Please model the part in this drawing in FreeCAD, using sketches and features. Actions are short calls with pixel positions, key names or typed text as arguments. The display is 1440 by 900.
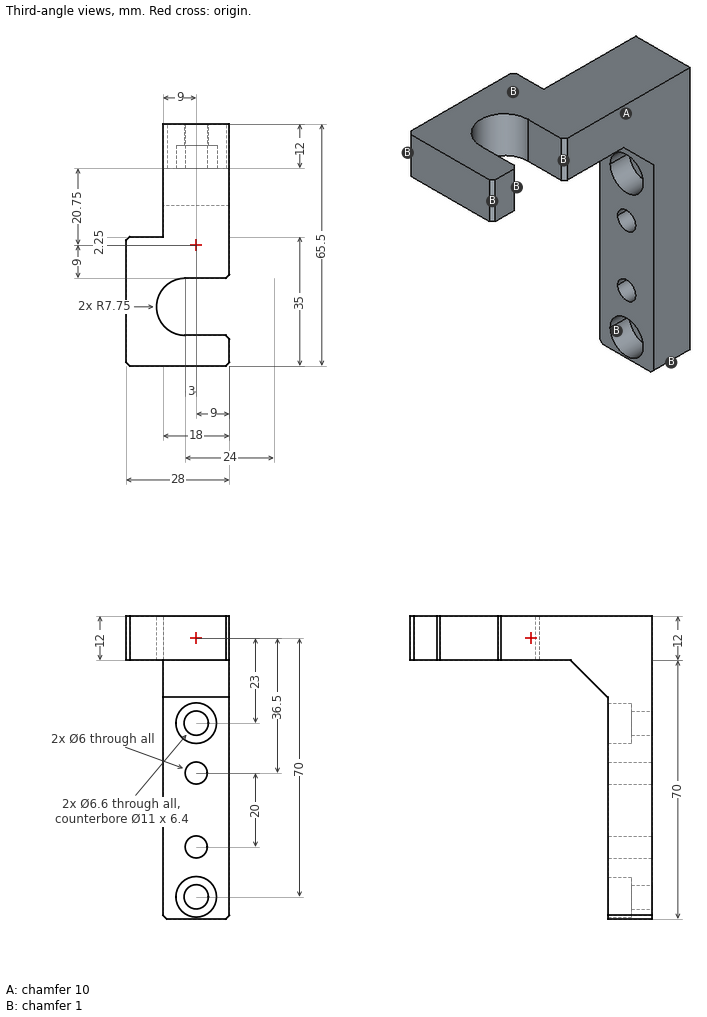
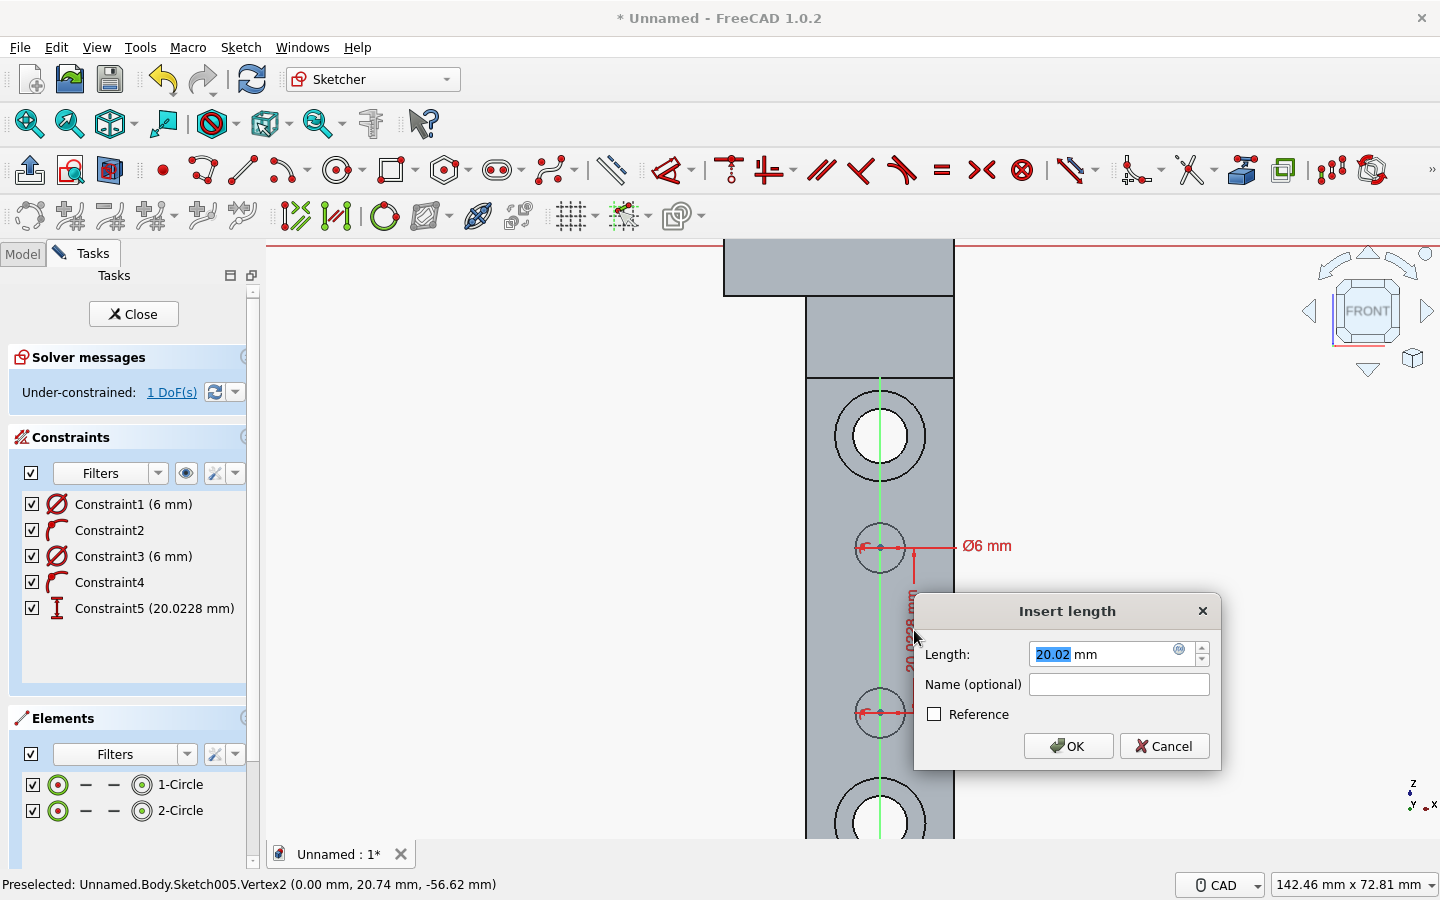
text(20)
key(Return)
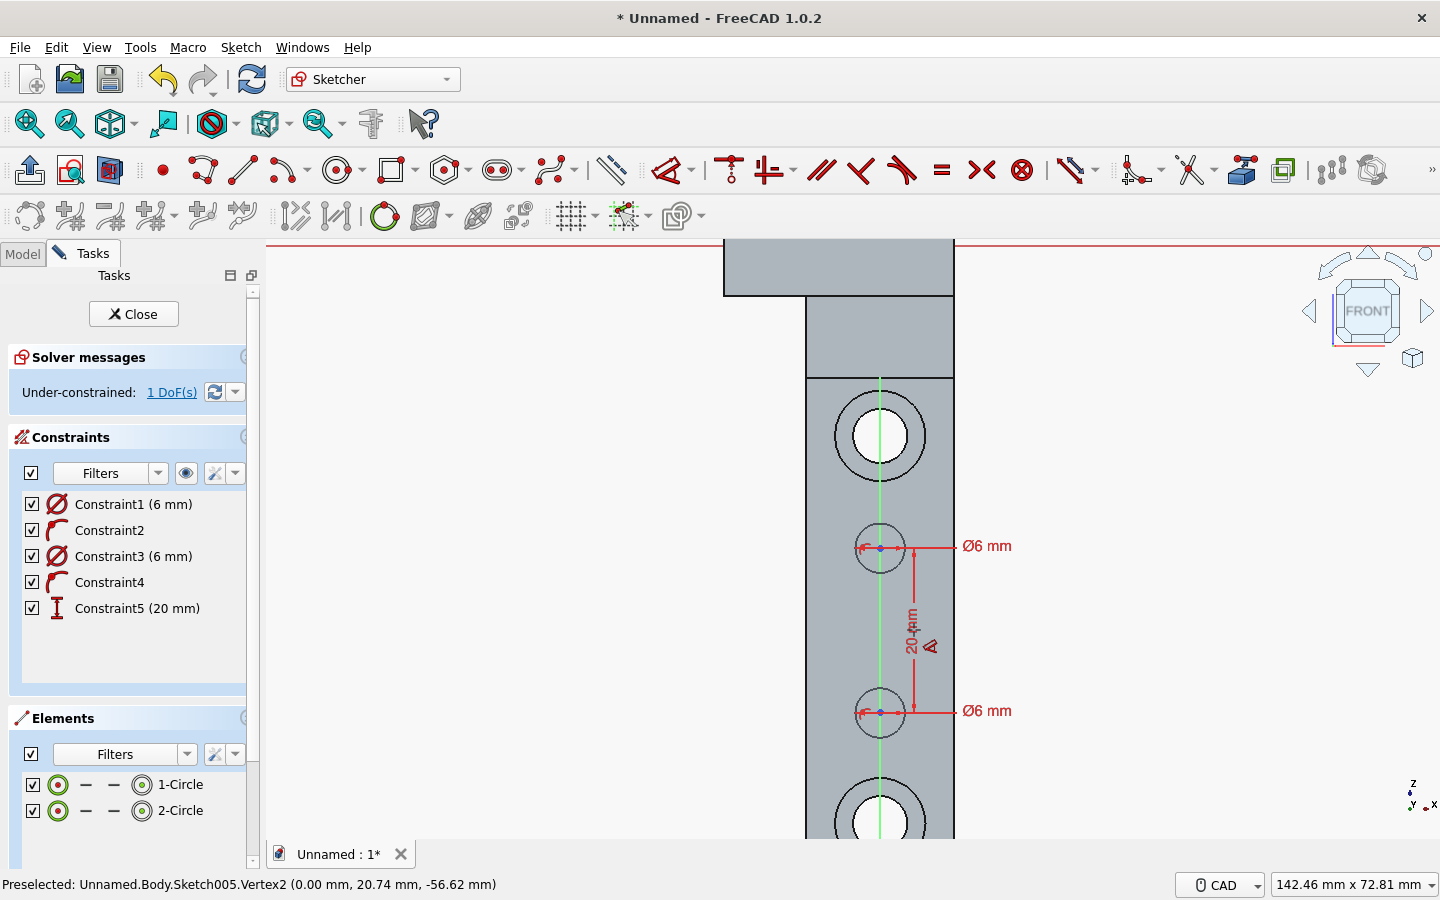
click(880, 548)
click(914, 408)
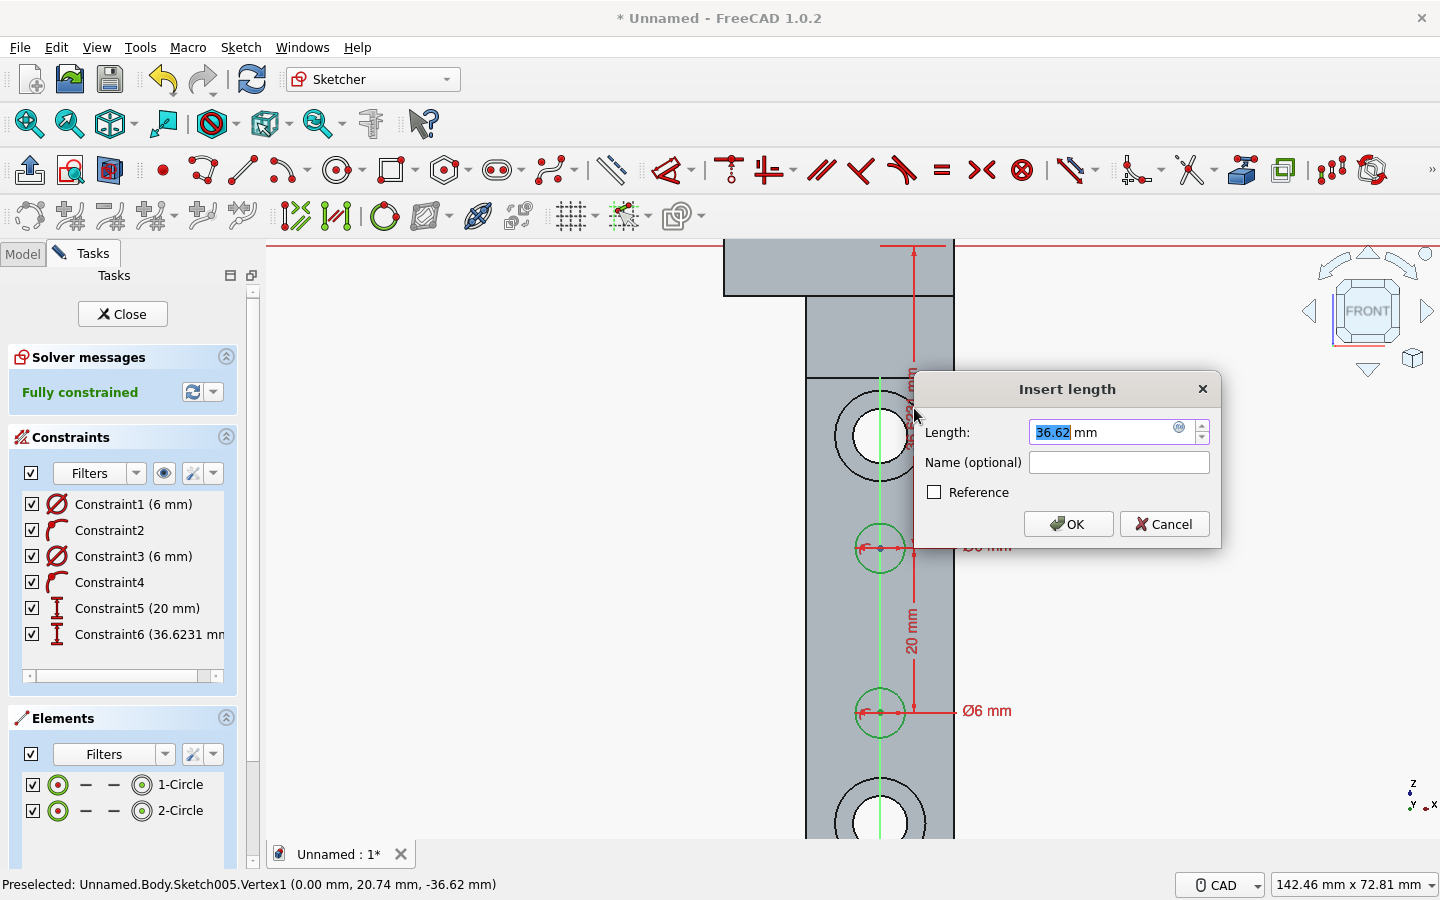
text(36.5)
key(Return)
key(Escape)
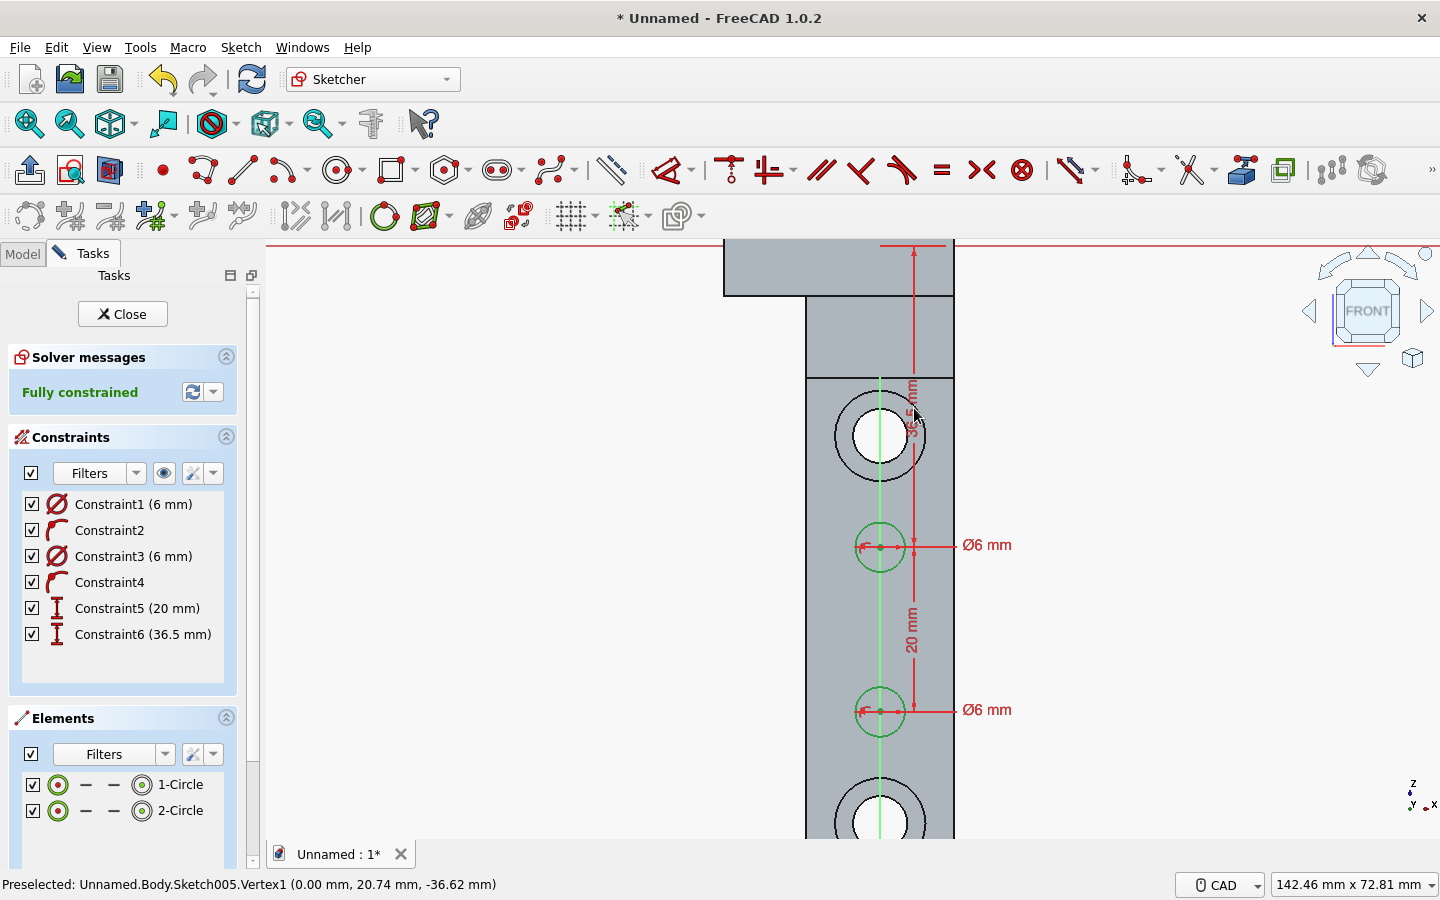
click(123, 314)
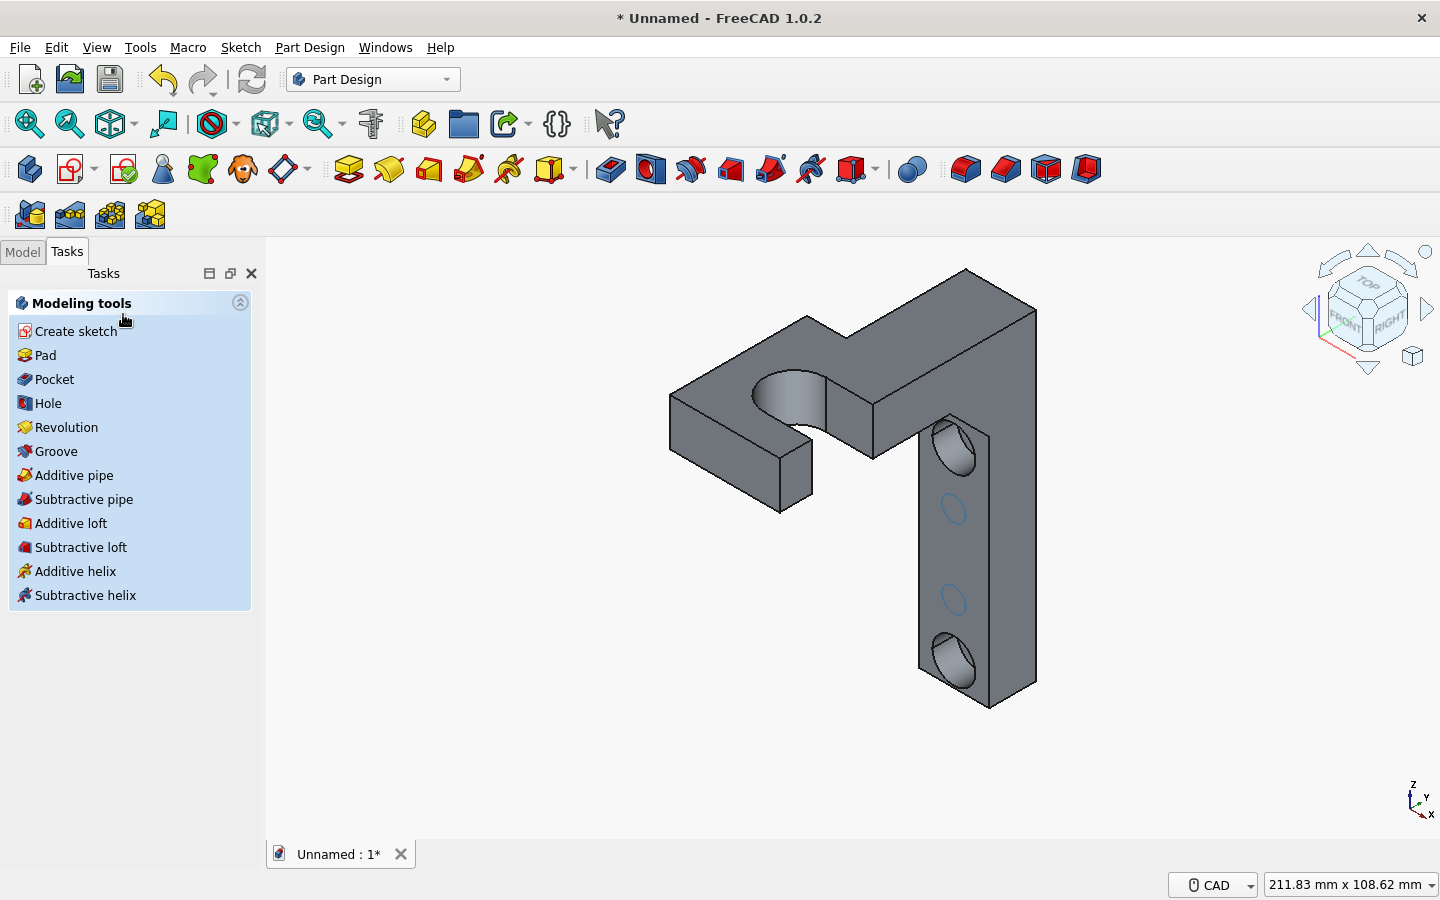
click(652, 170)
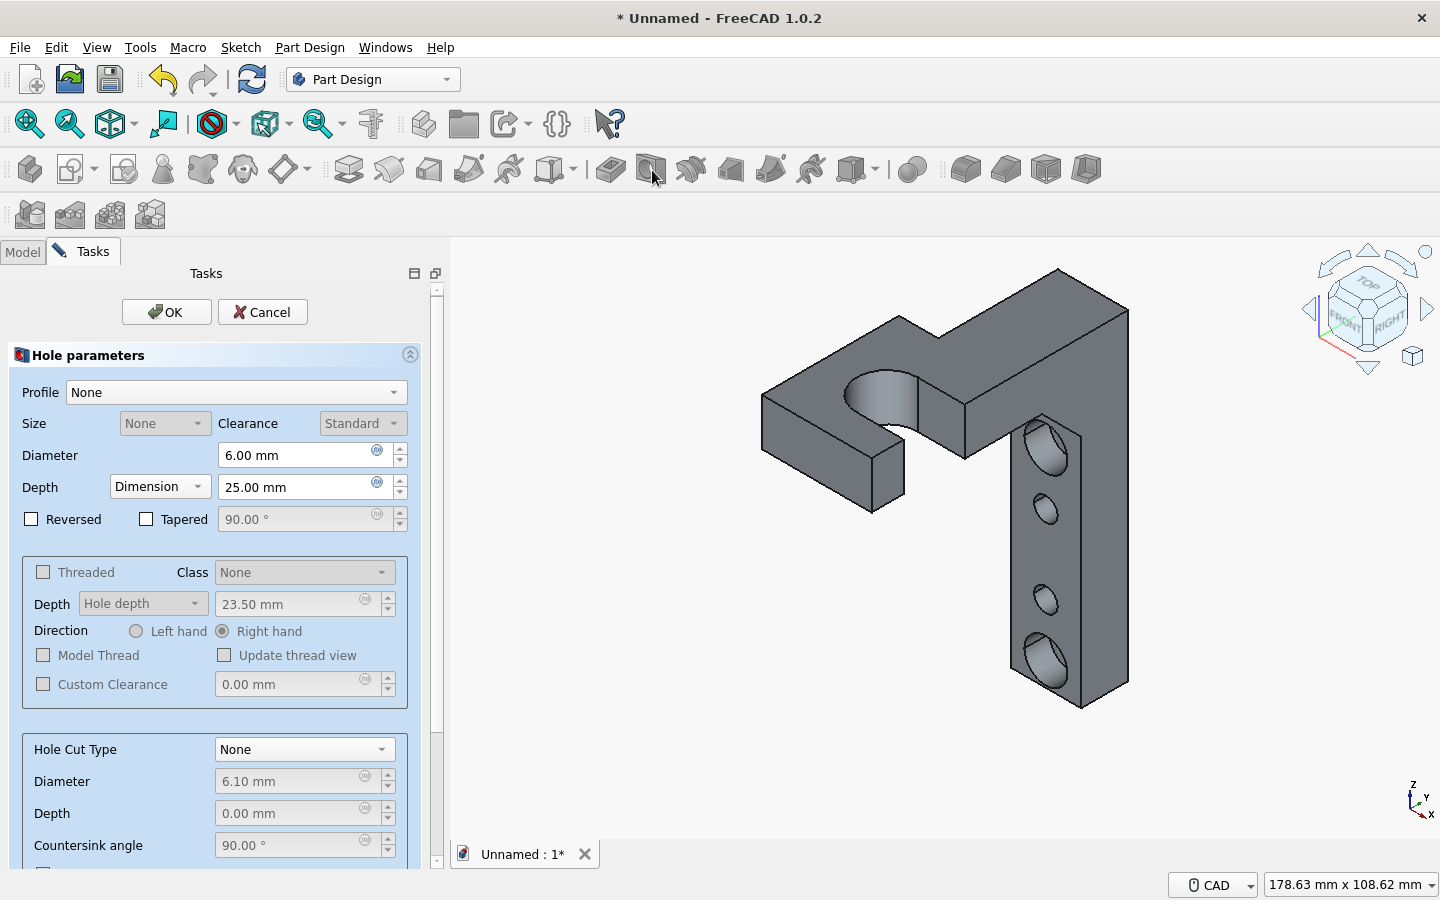
triple_click(305, 455)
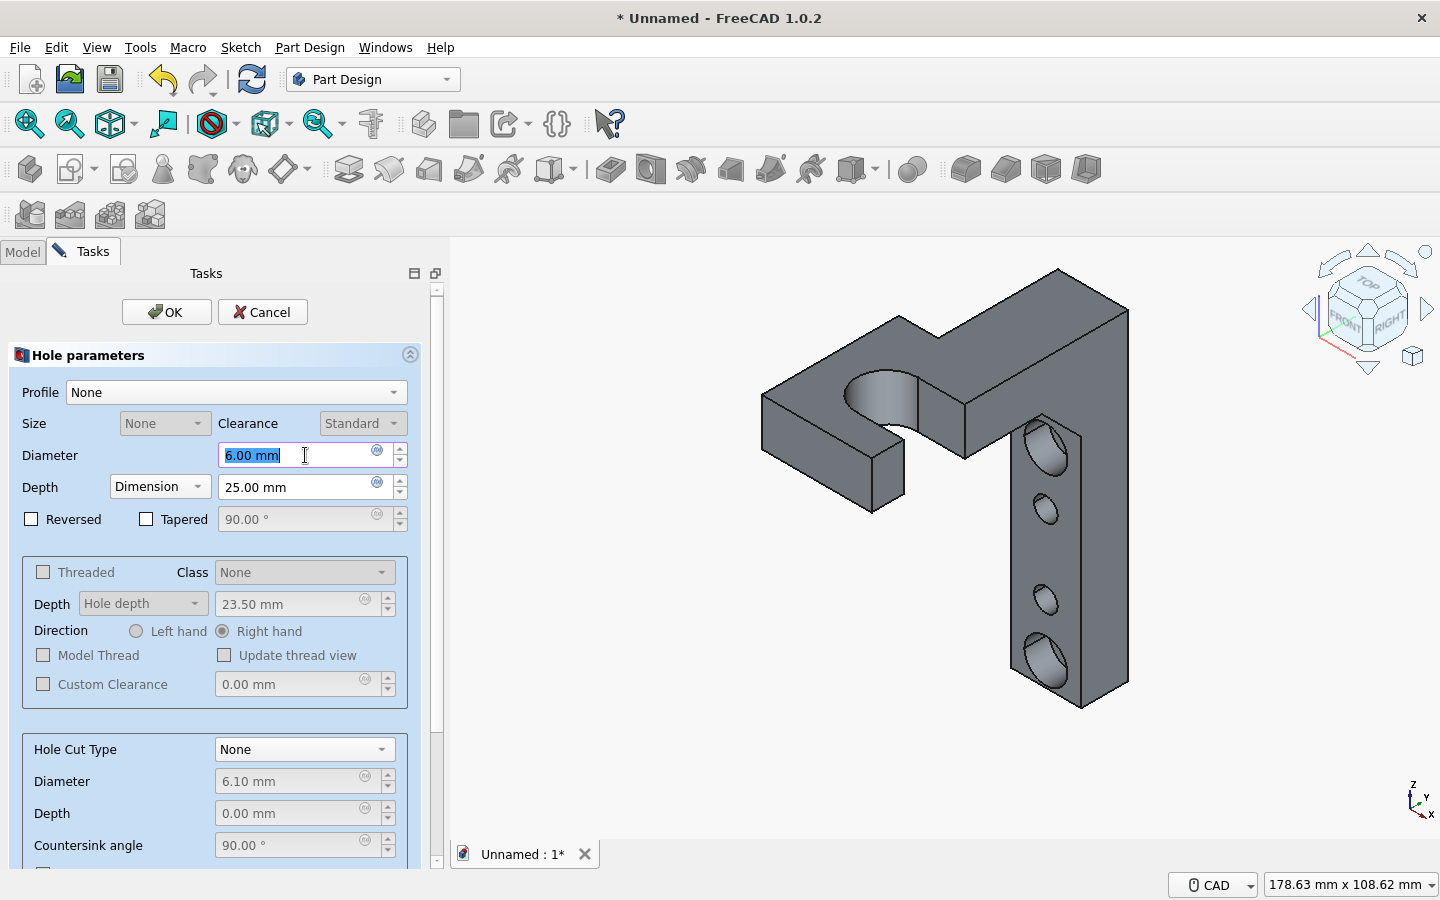
text(6)
key(Tab)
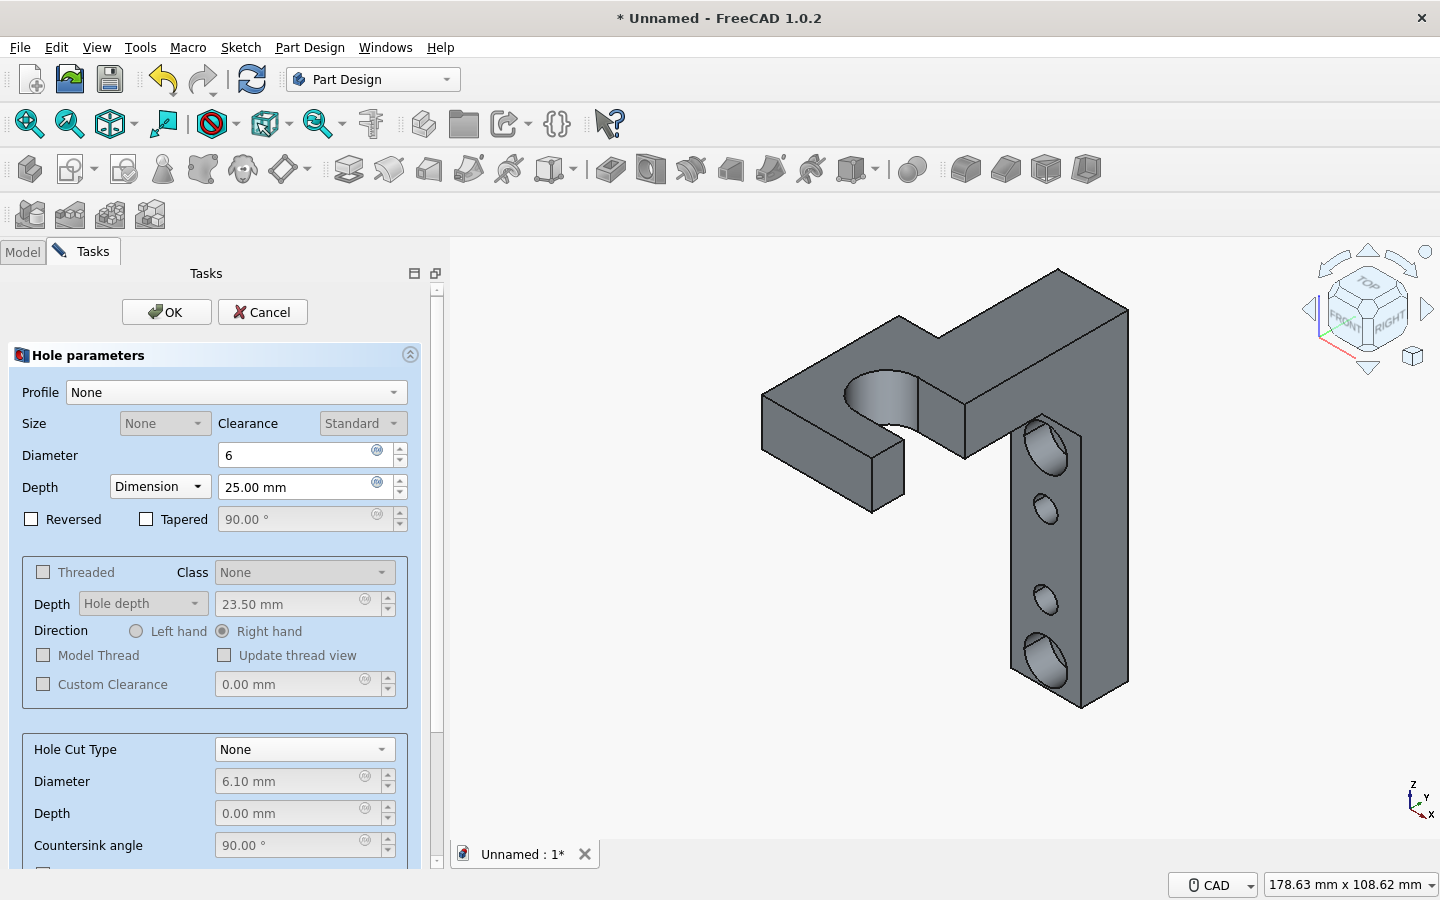
click(161, 486)